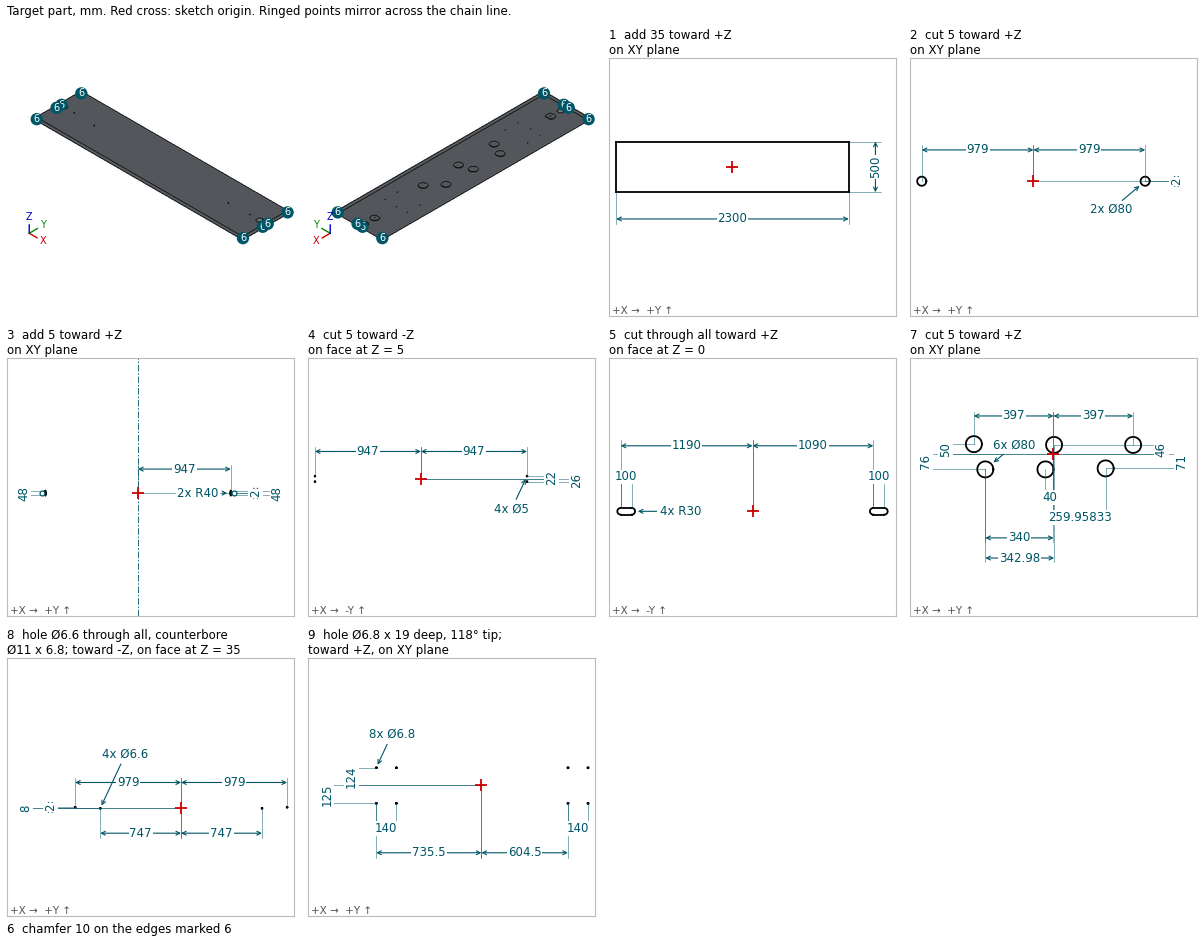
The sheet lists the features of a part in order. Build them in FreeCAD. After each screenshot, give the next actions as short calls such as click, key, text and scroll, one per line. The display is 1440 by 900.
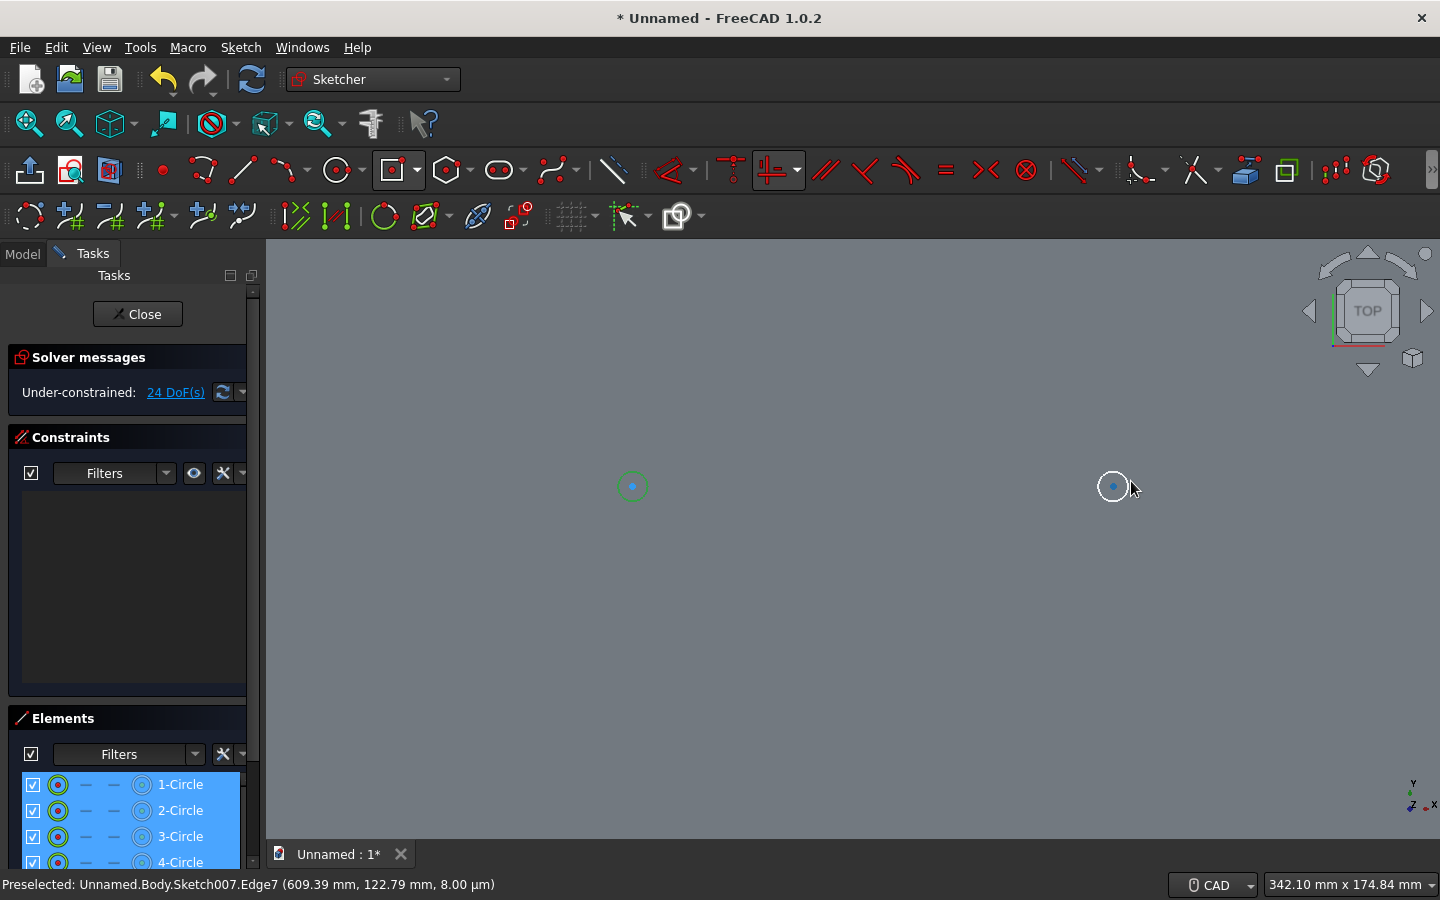
click(1124, 476)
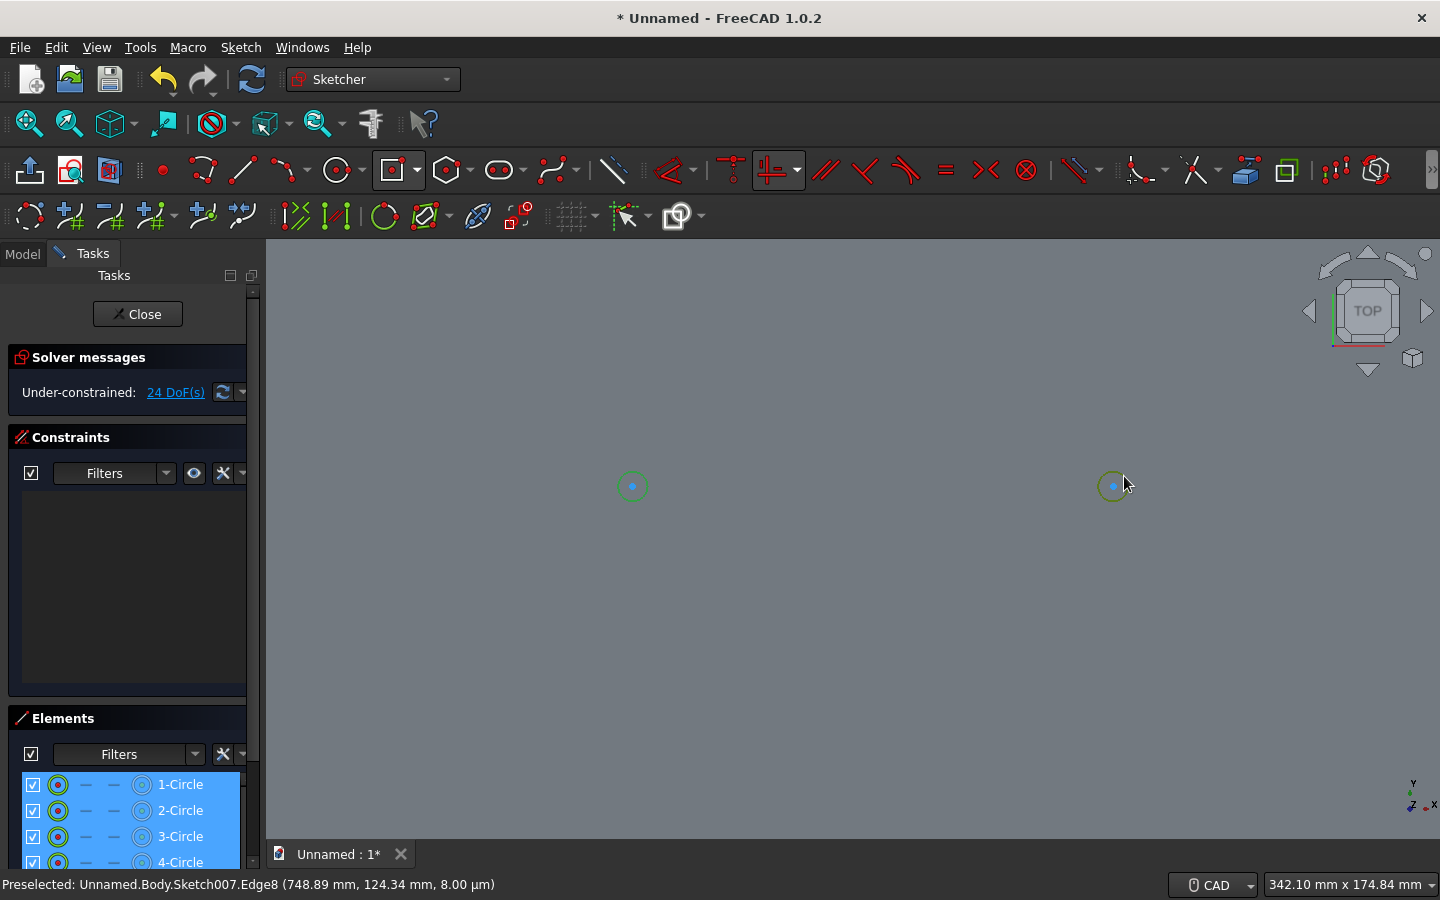
click(946, 170)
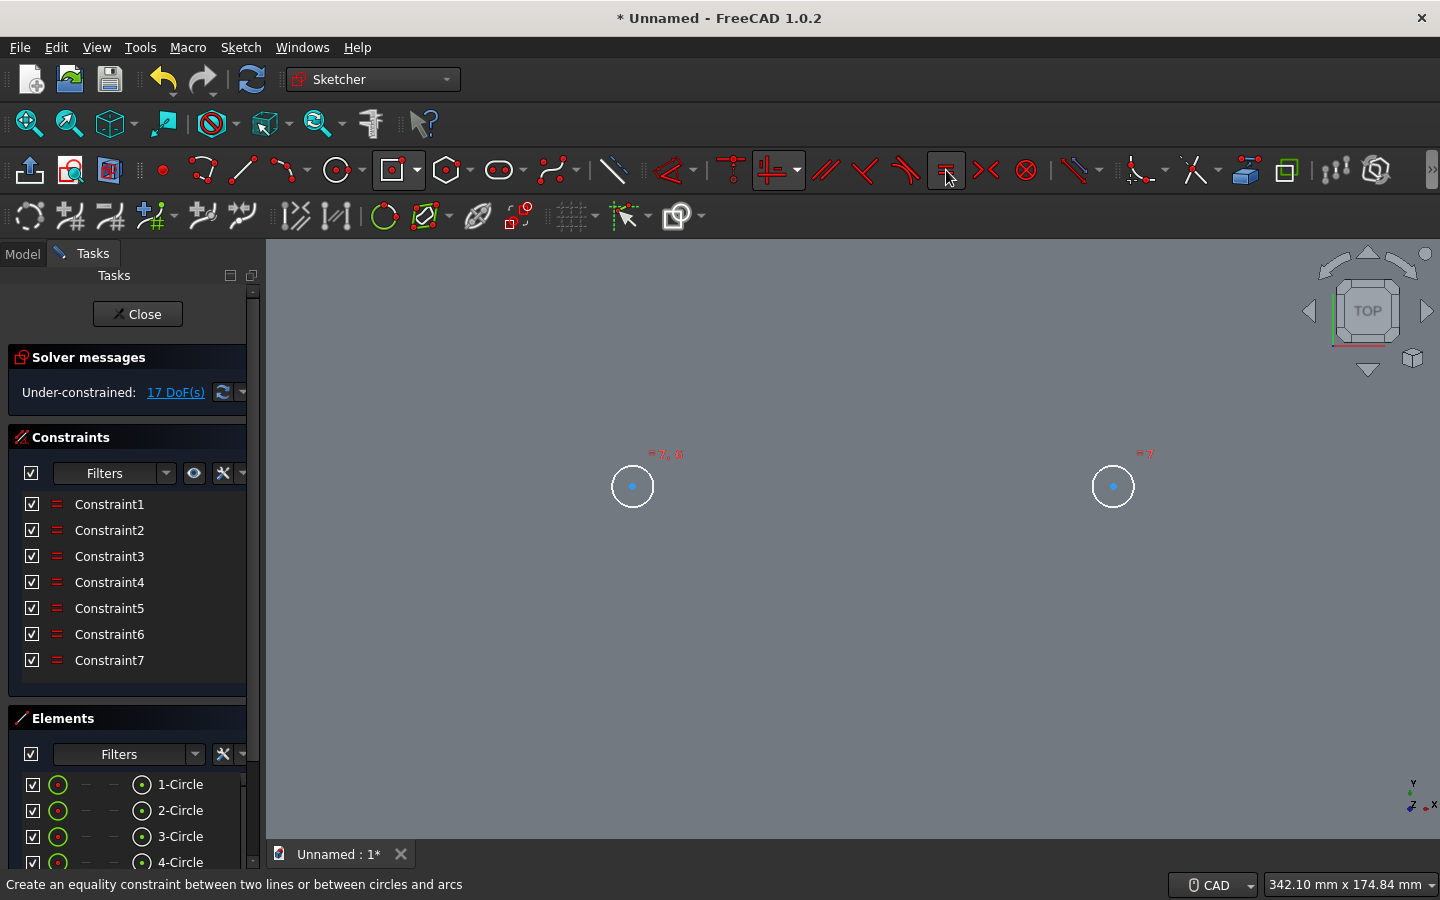
scroll(1131, 481, down, 10)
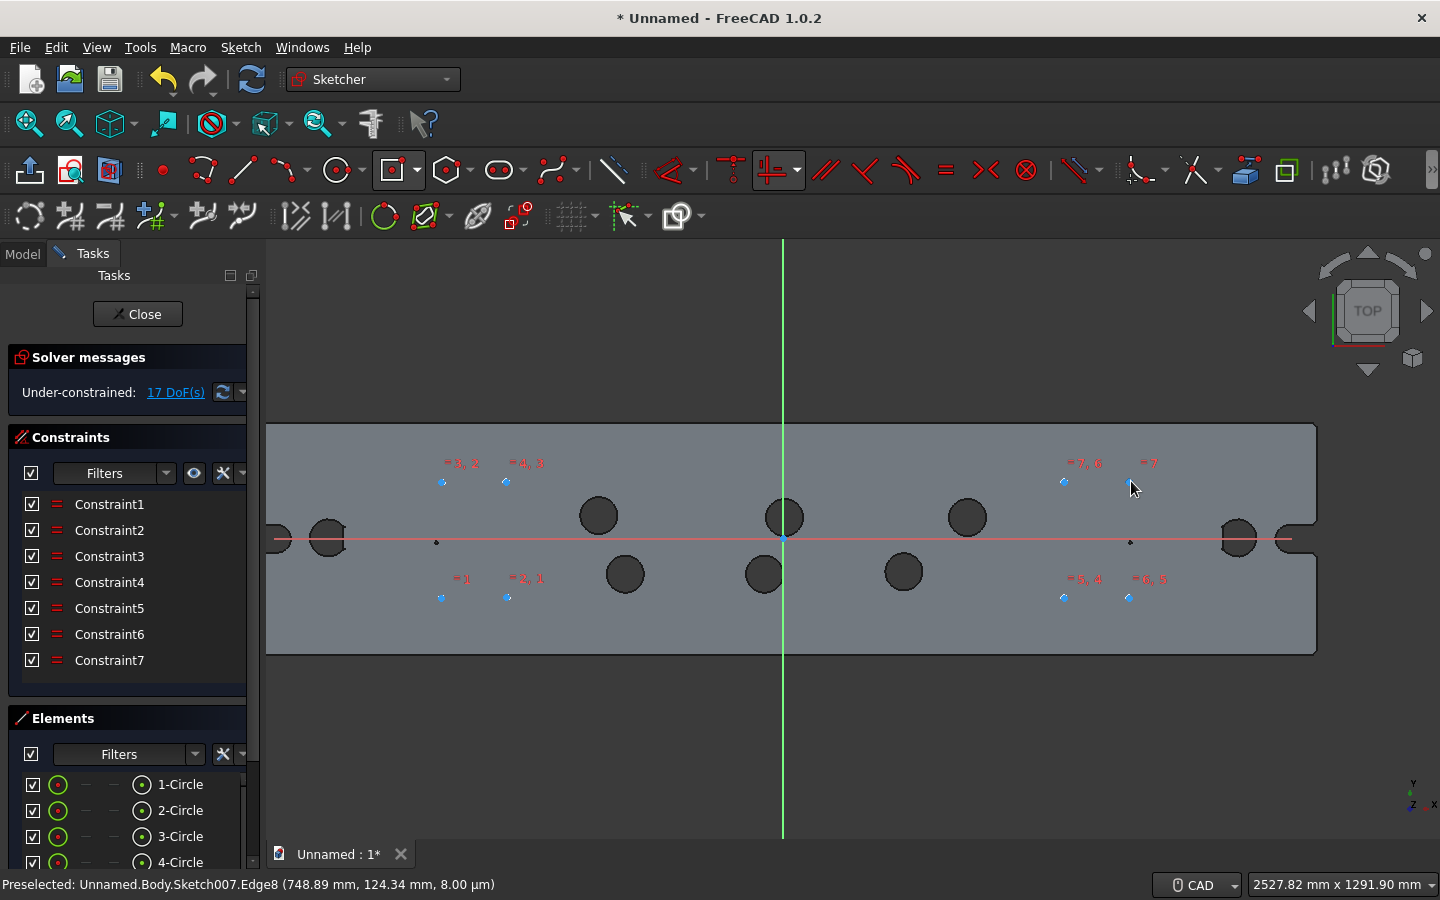
click(441, 598)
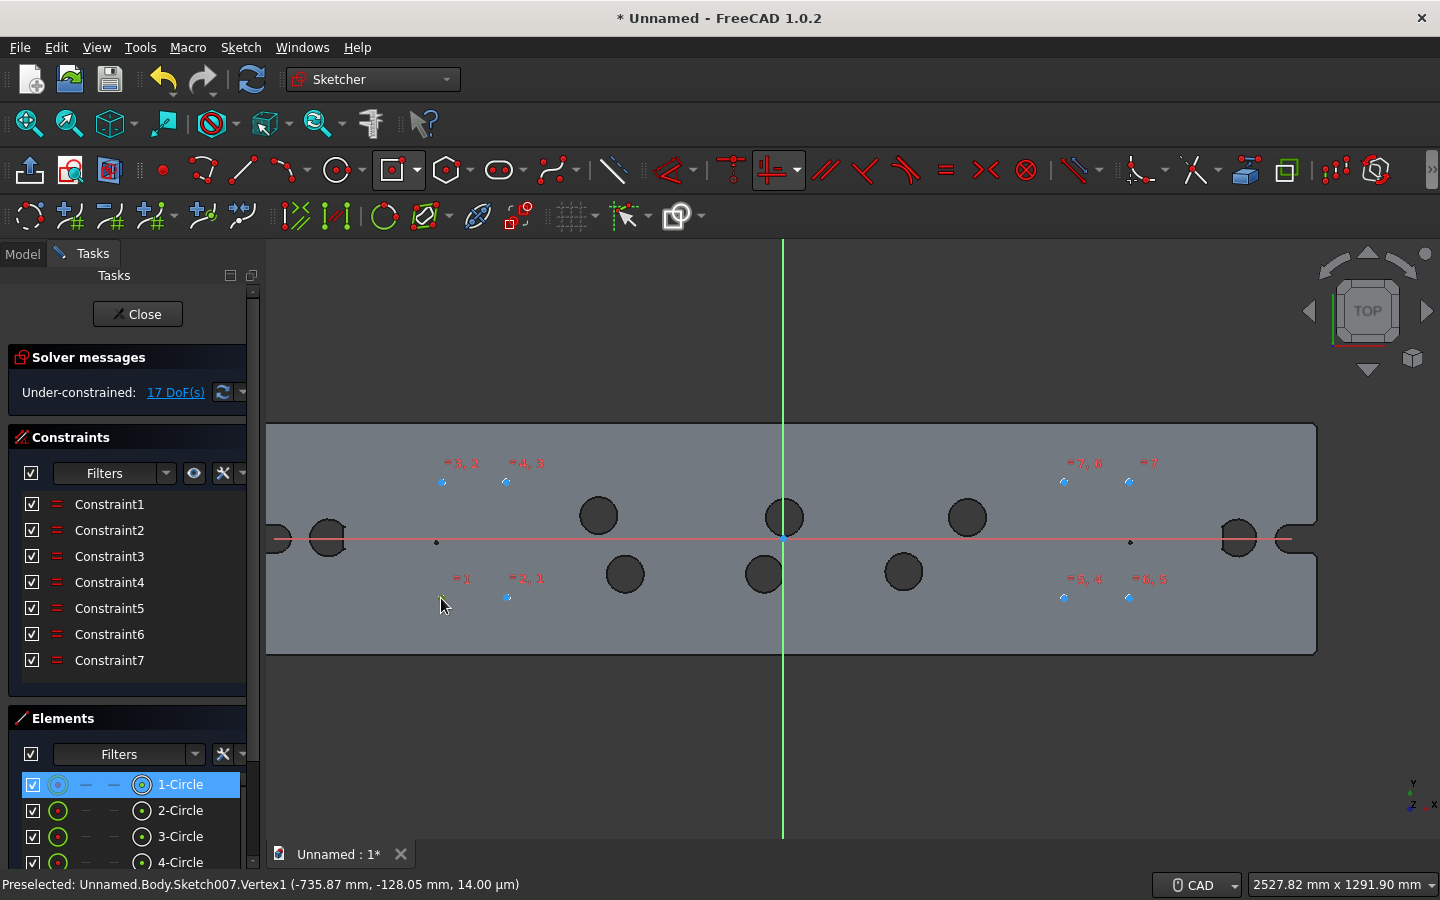
click(507, 598)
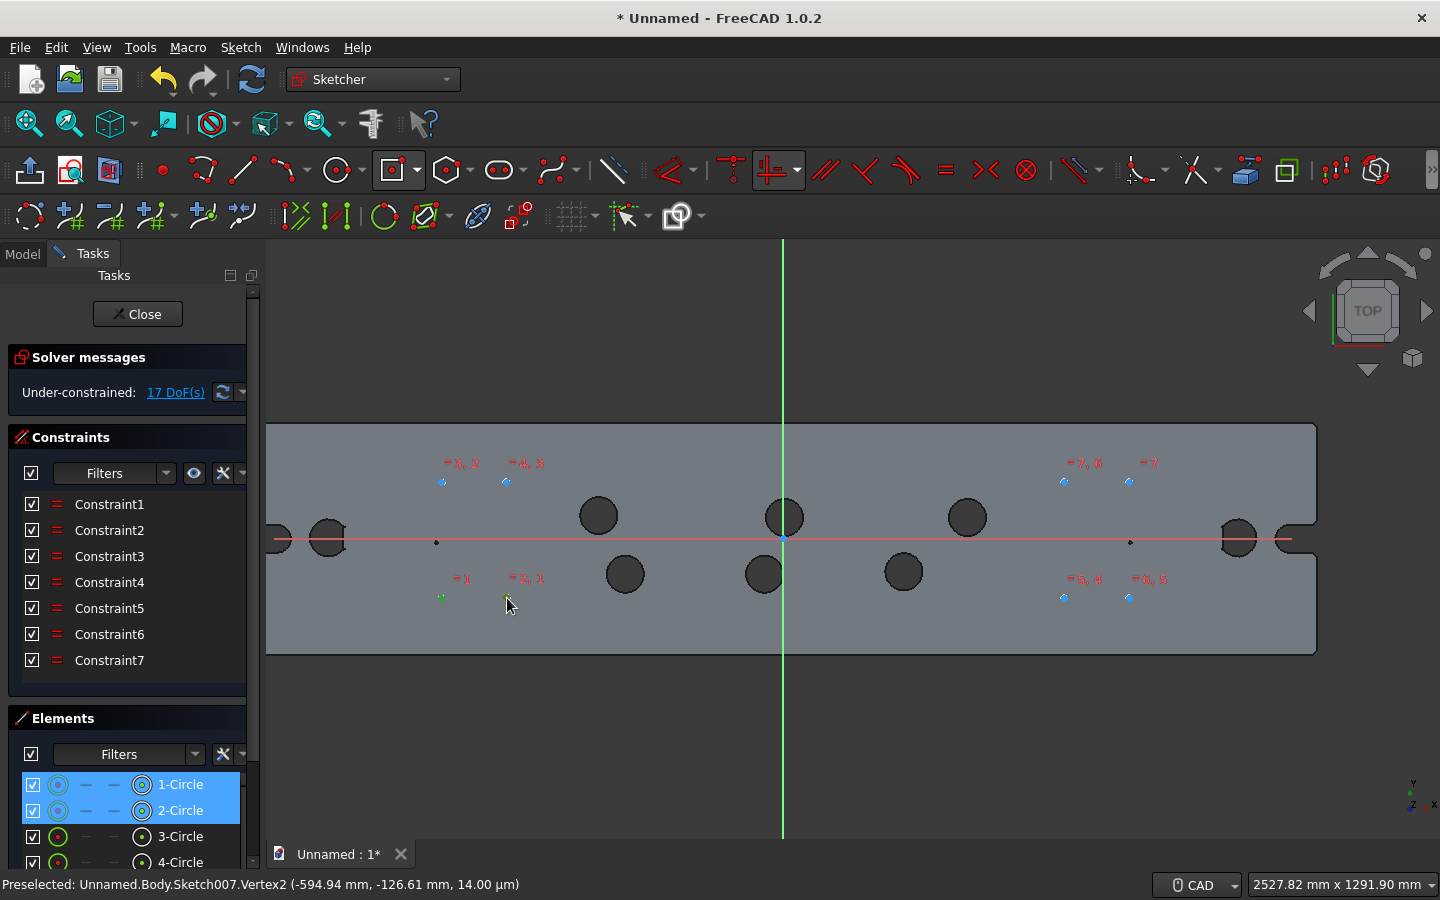
key(h)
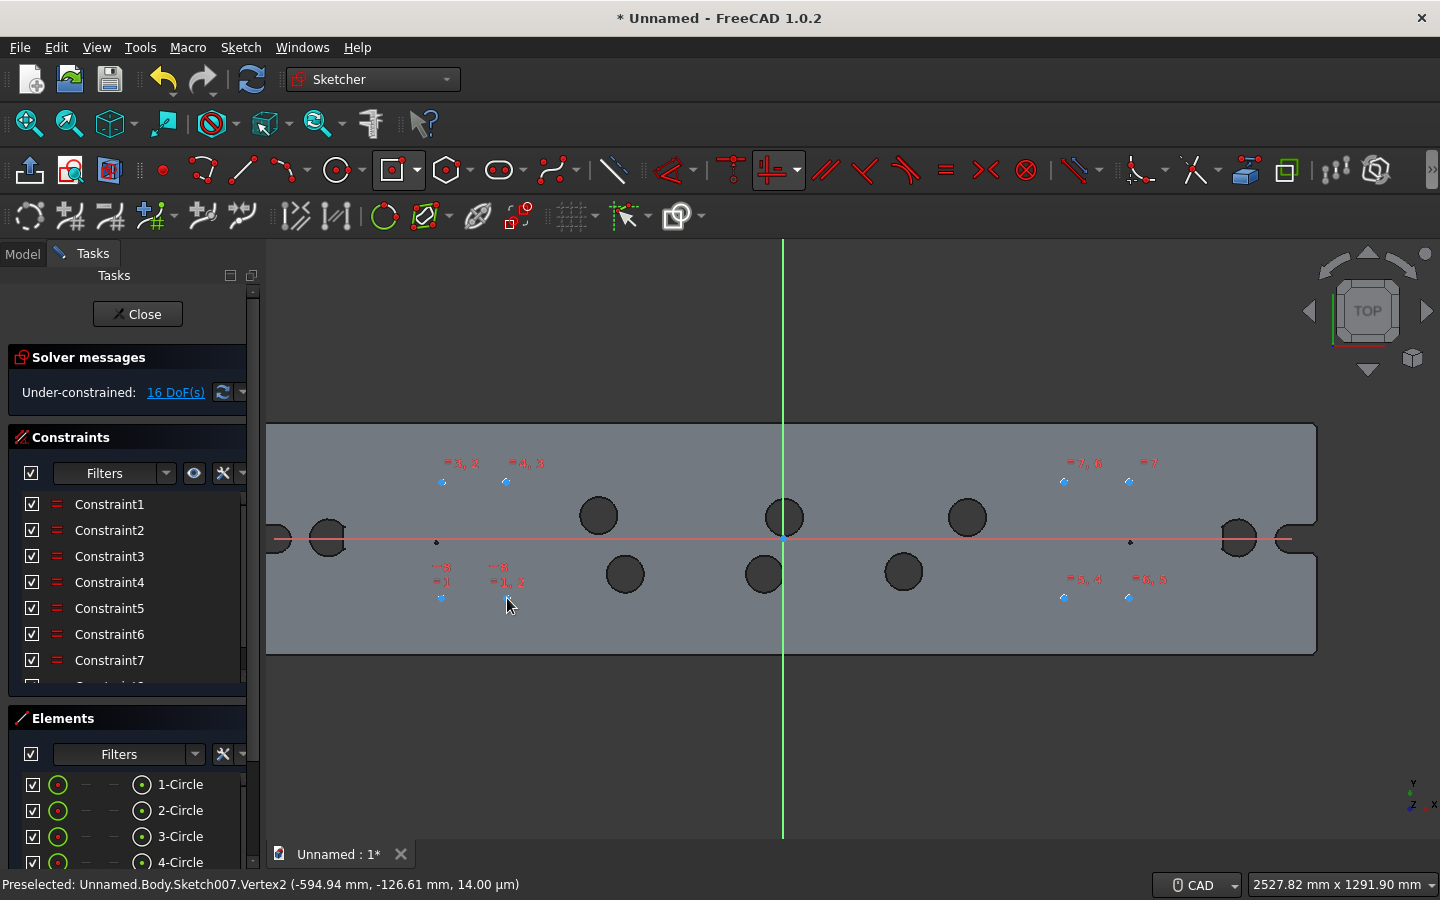
click(441, 598)